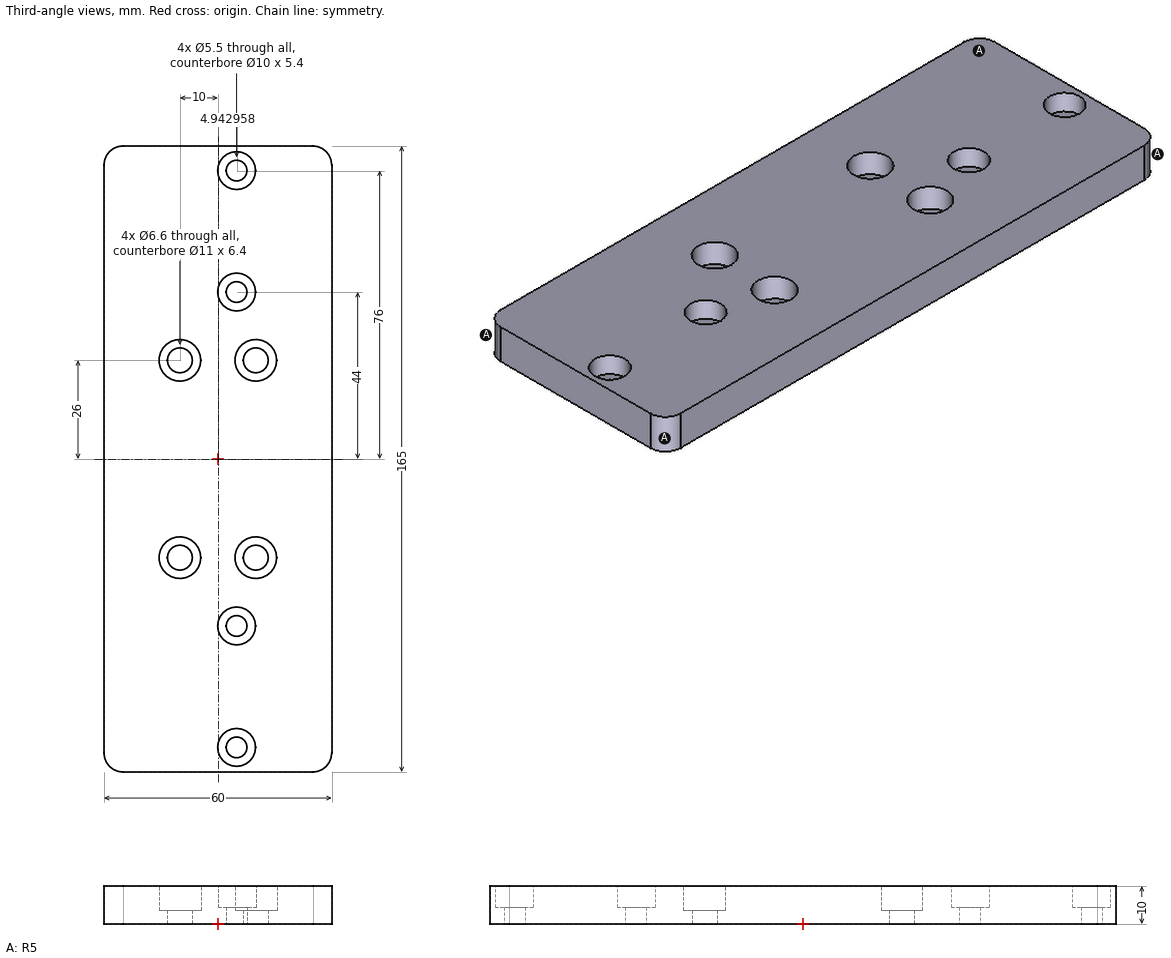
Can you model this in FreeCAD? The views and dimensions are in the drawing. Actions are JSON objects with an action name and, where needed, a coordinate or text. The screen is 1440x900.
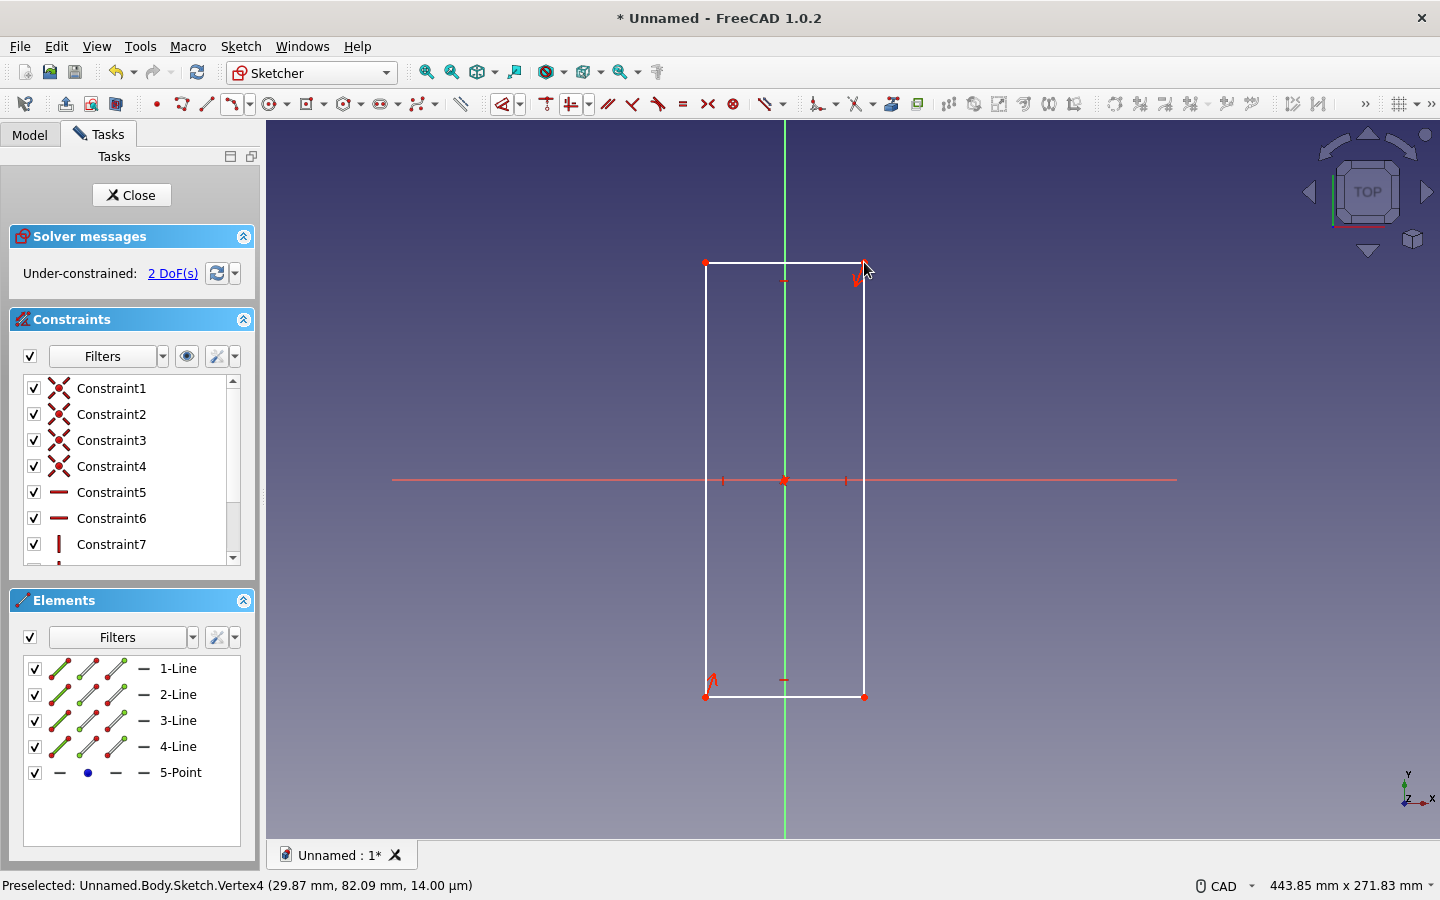
{"action": "left_click", "coordinate": [502, 104]}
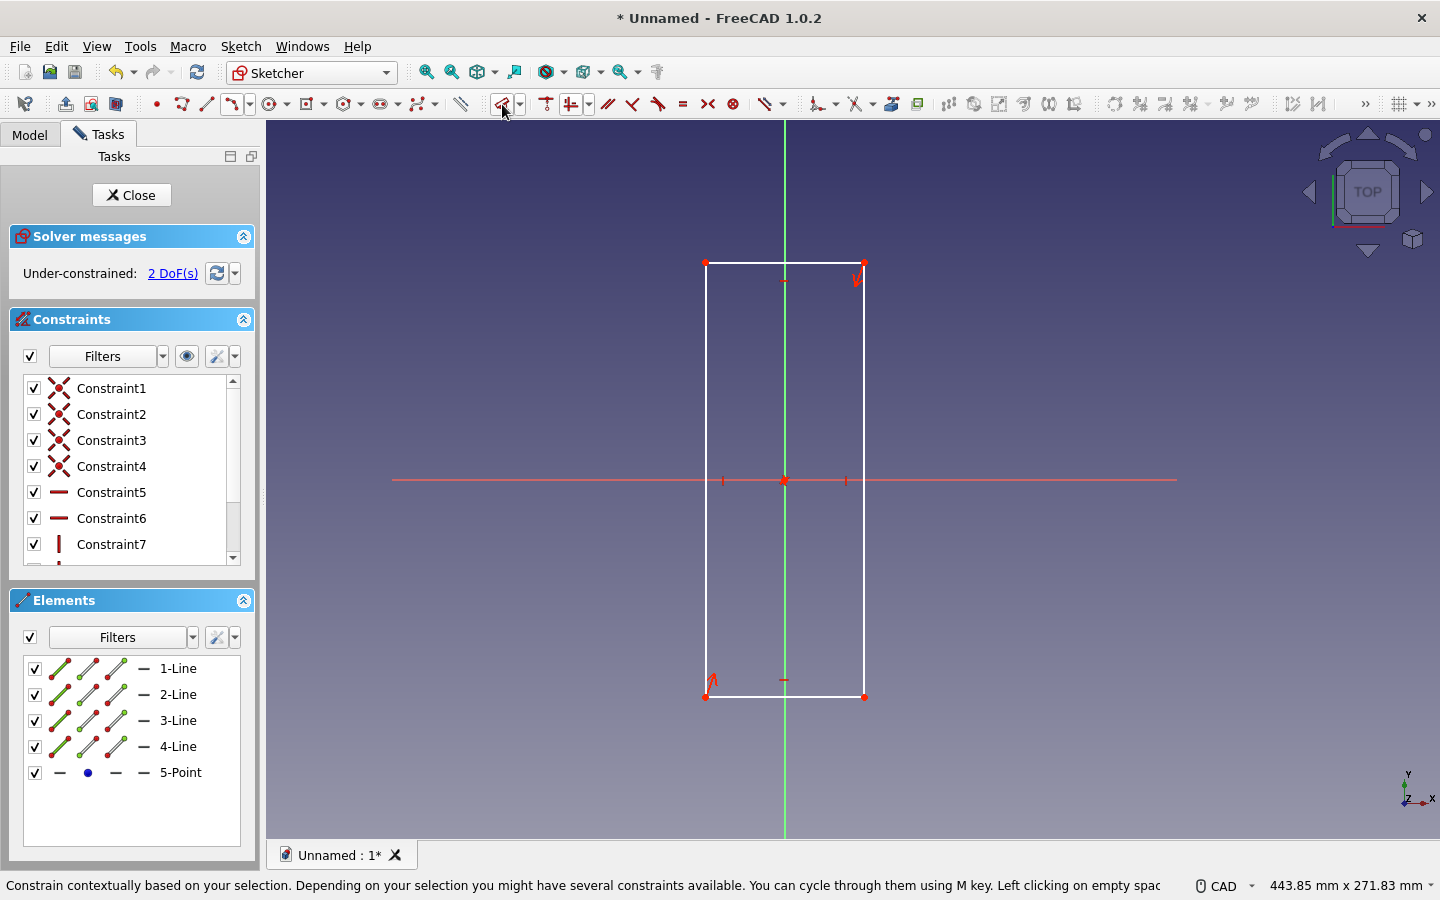
{"action": "left_click", "coordinate": [753, 697]}
{"action": "left_click", "coordinate": [749, 731]}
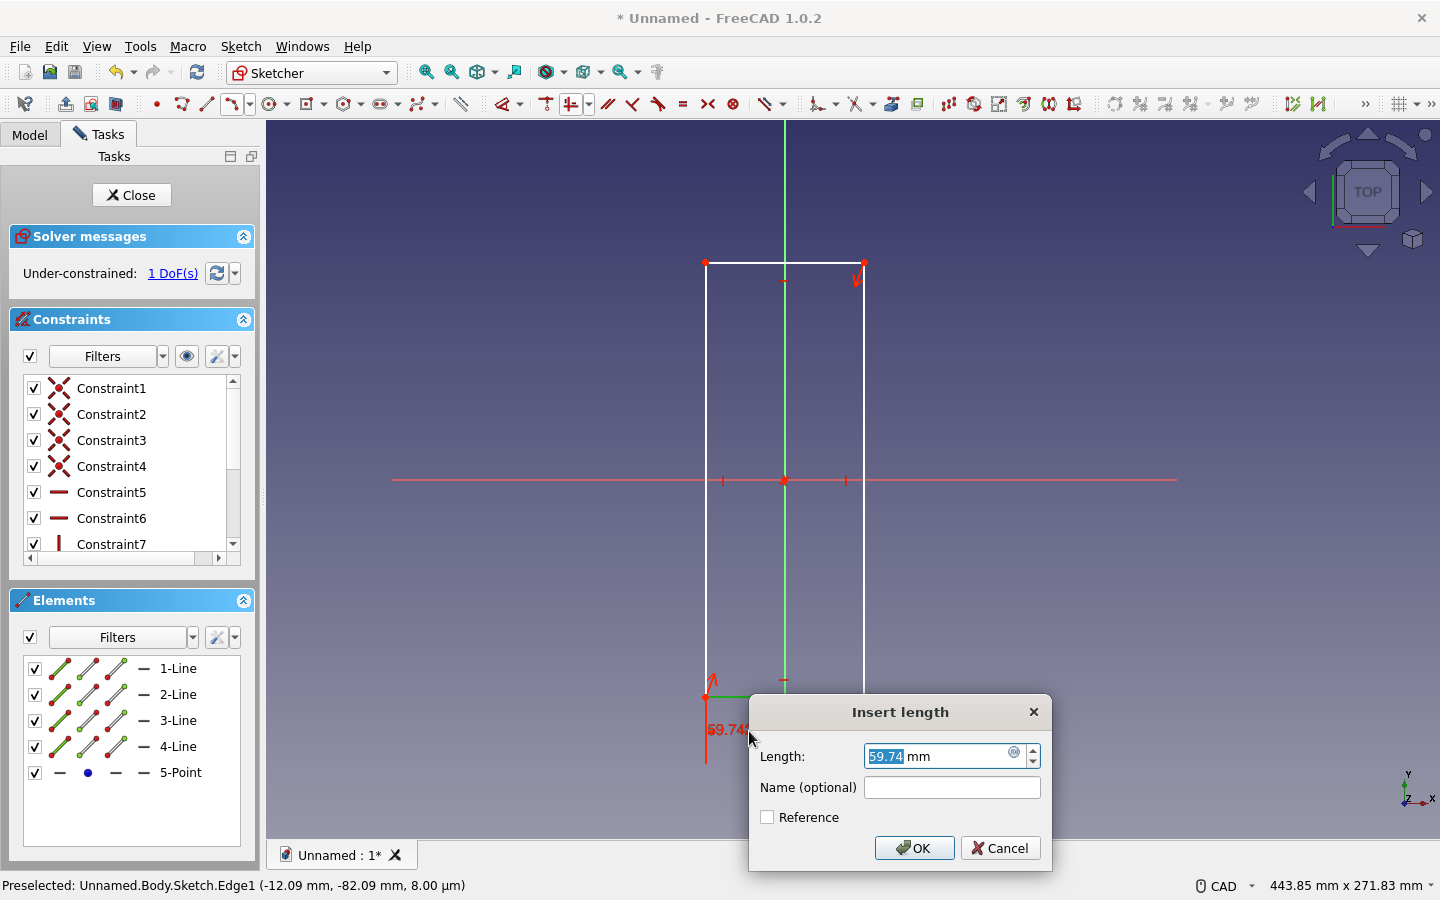
{"action": "type", "text": "60"}
{"action": "key", "text": "Return"}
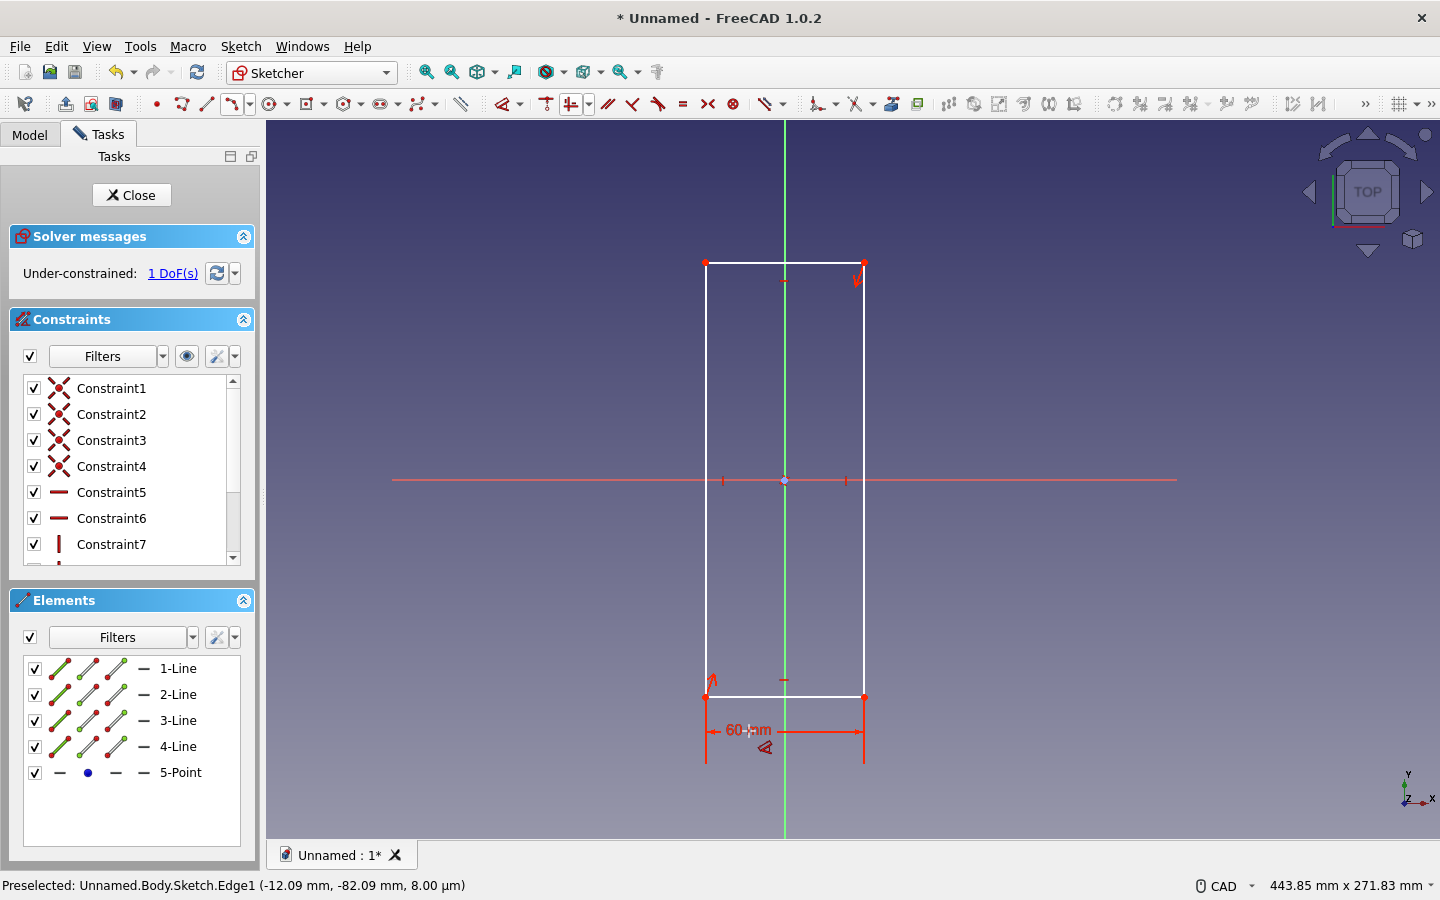
{"action": "left_click", "coordinate": [864, 567]}
{"action": "left_click", "coordinate": [898, 380]}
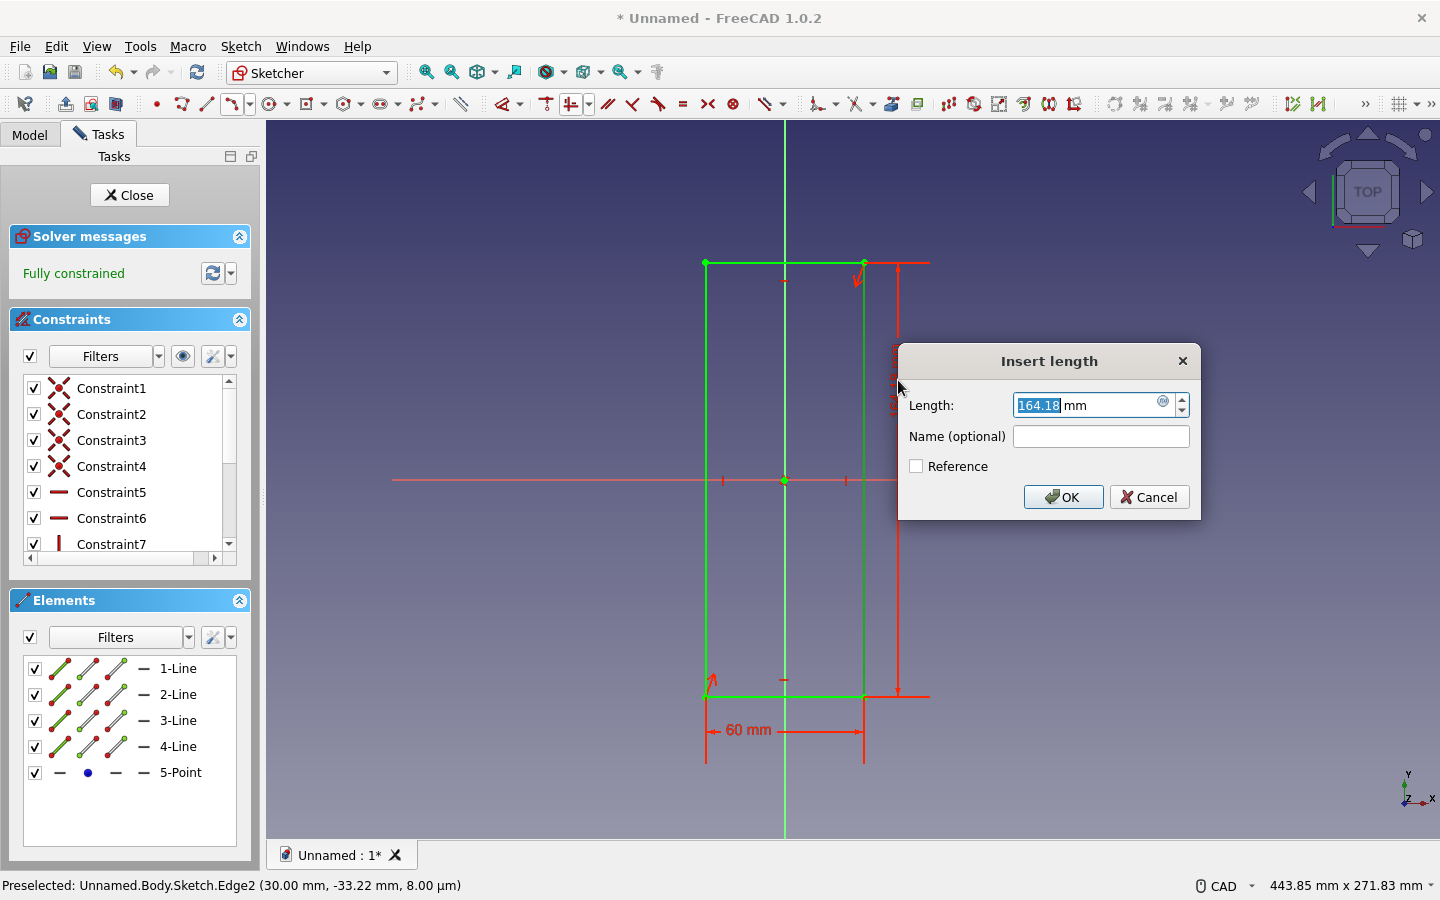
{"action": "type", "text": "165"}
{"action": "key", "text": "Return"}
{"action": "key", "text": "Escape"}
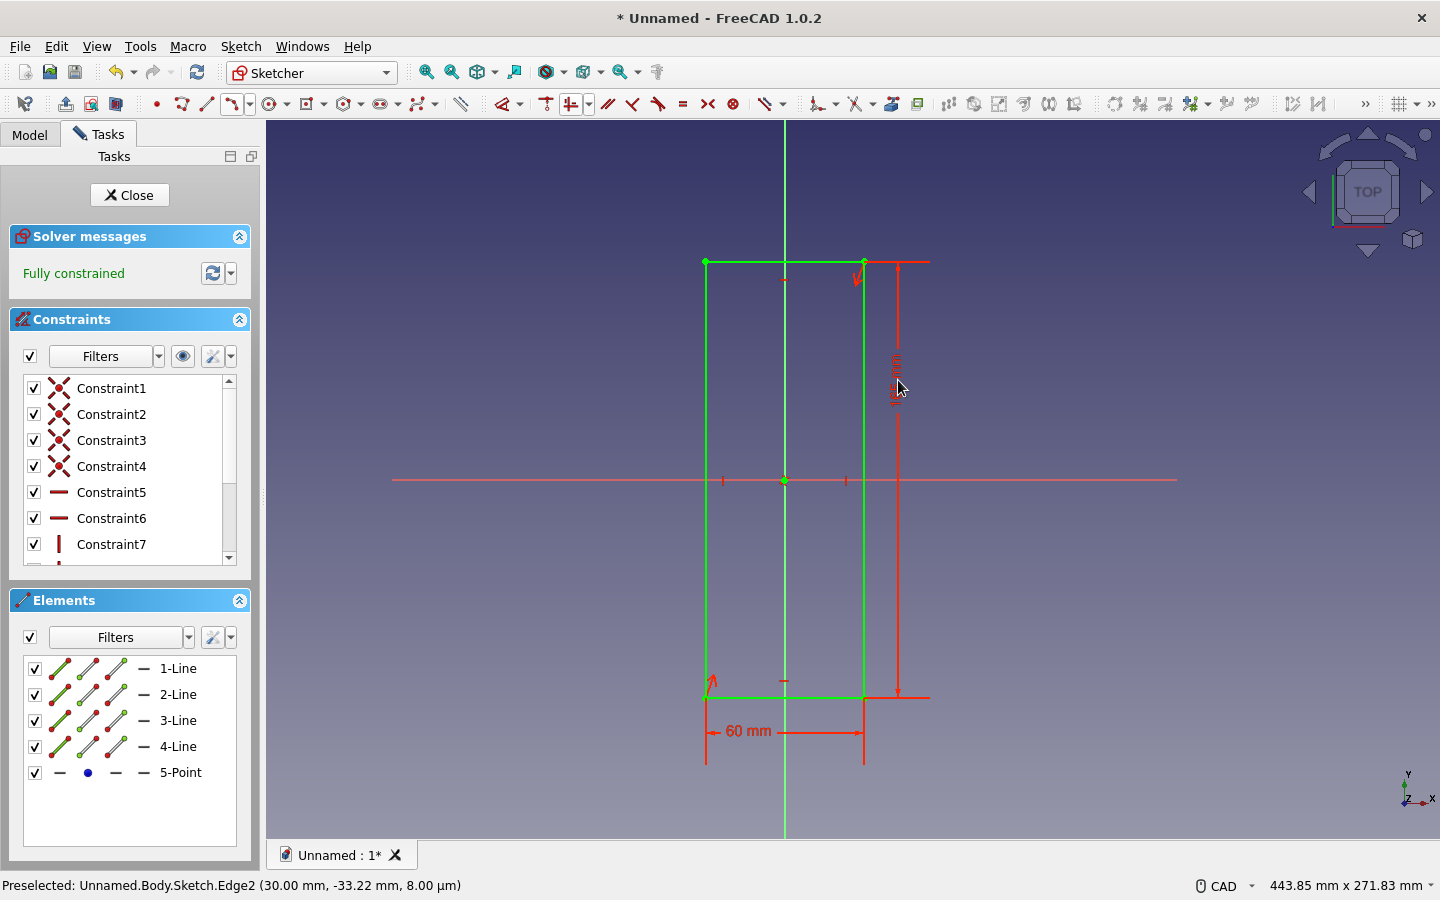
{"action": "left_click", "coordinate": [130, 195]}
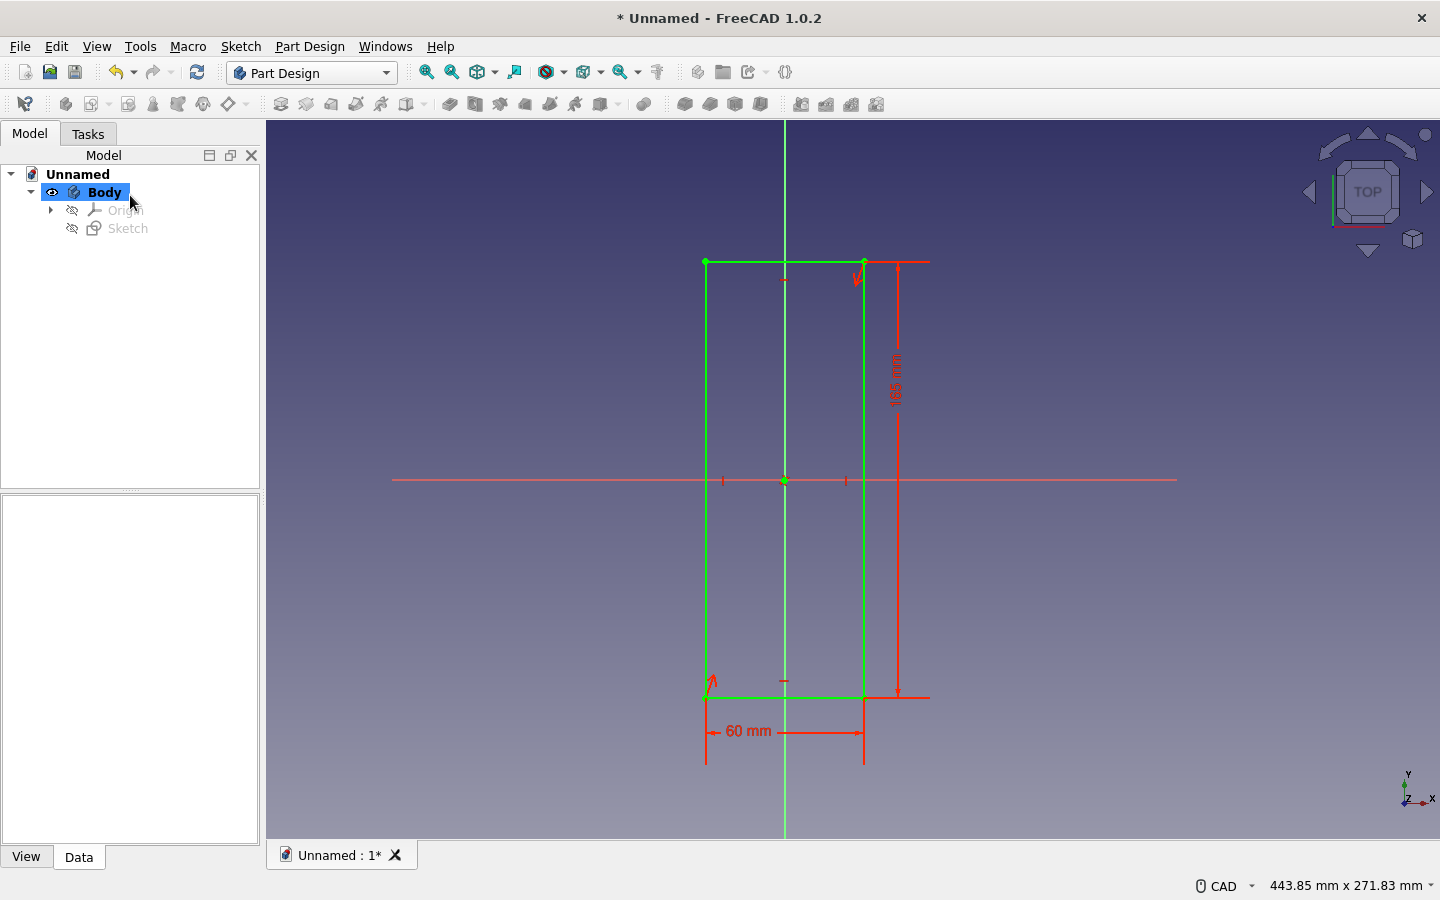
{"action": "left_click", "coordinate": [281, 104]}